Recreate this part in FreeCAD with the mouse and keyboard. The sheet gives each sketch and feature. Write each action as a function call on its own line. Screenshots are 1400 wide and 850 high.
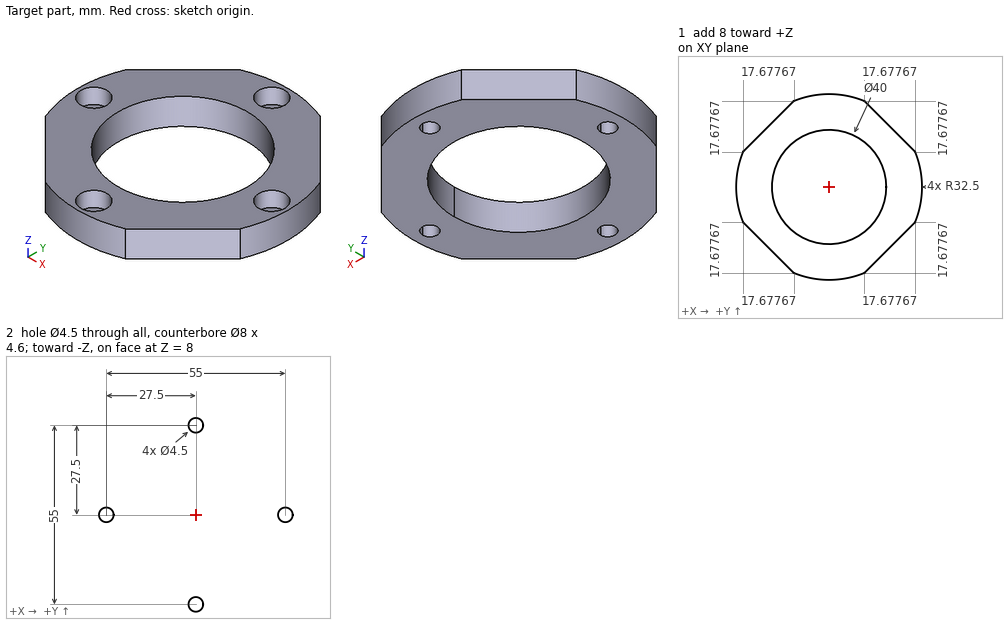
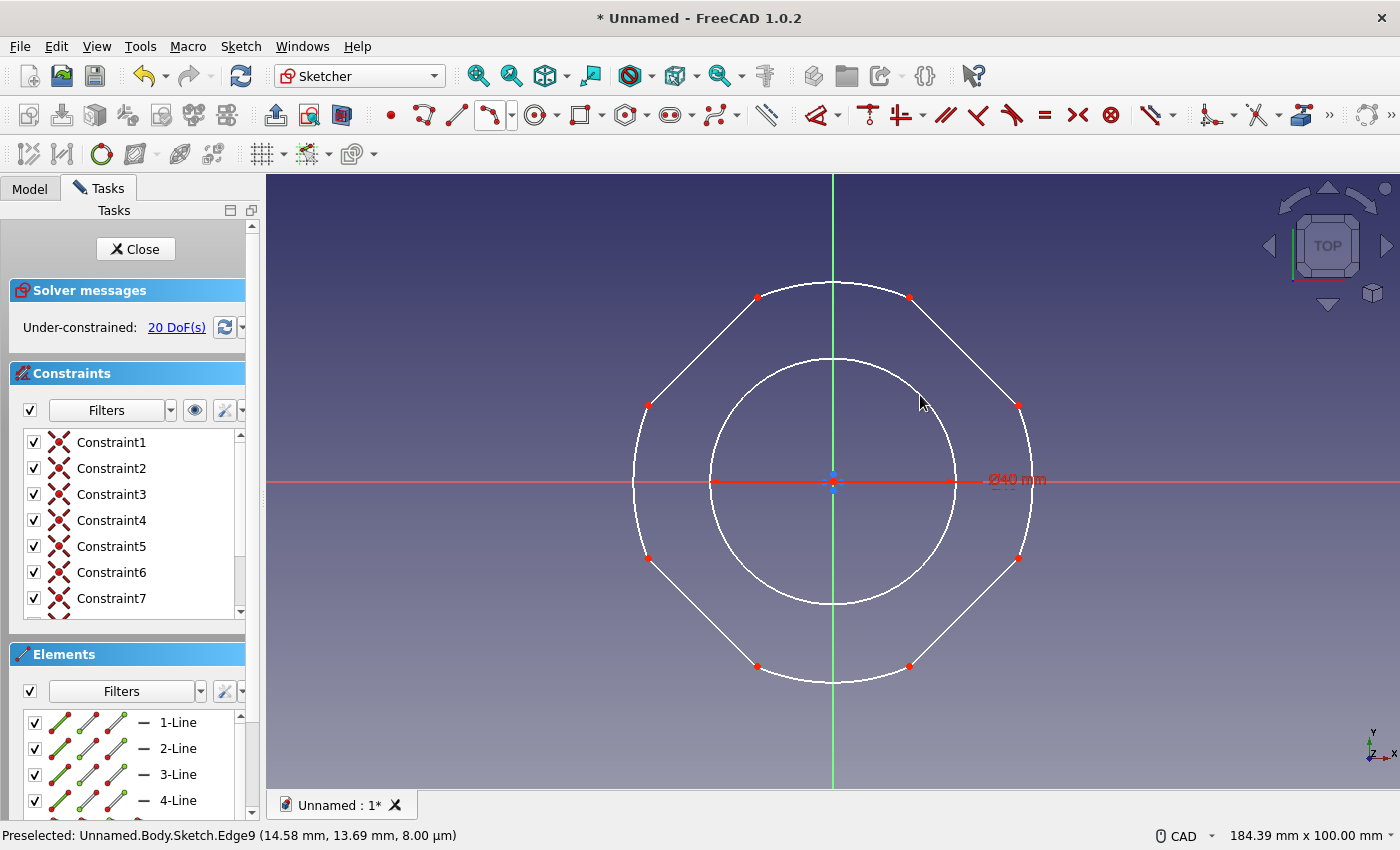
click(920, 394)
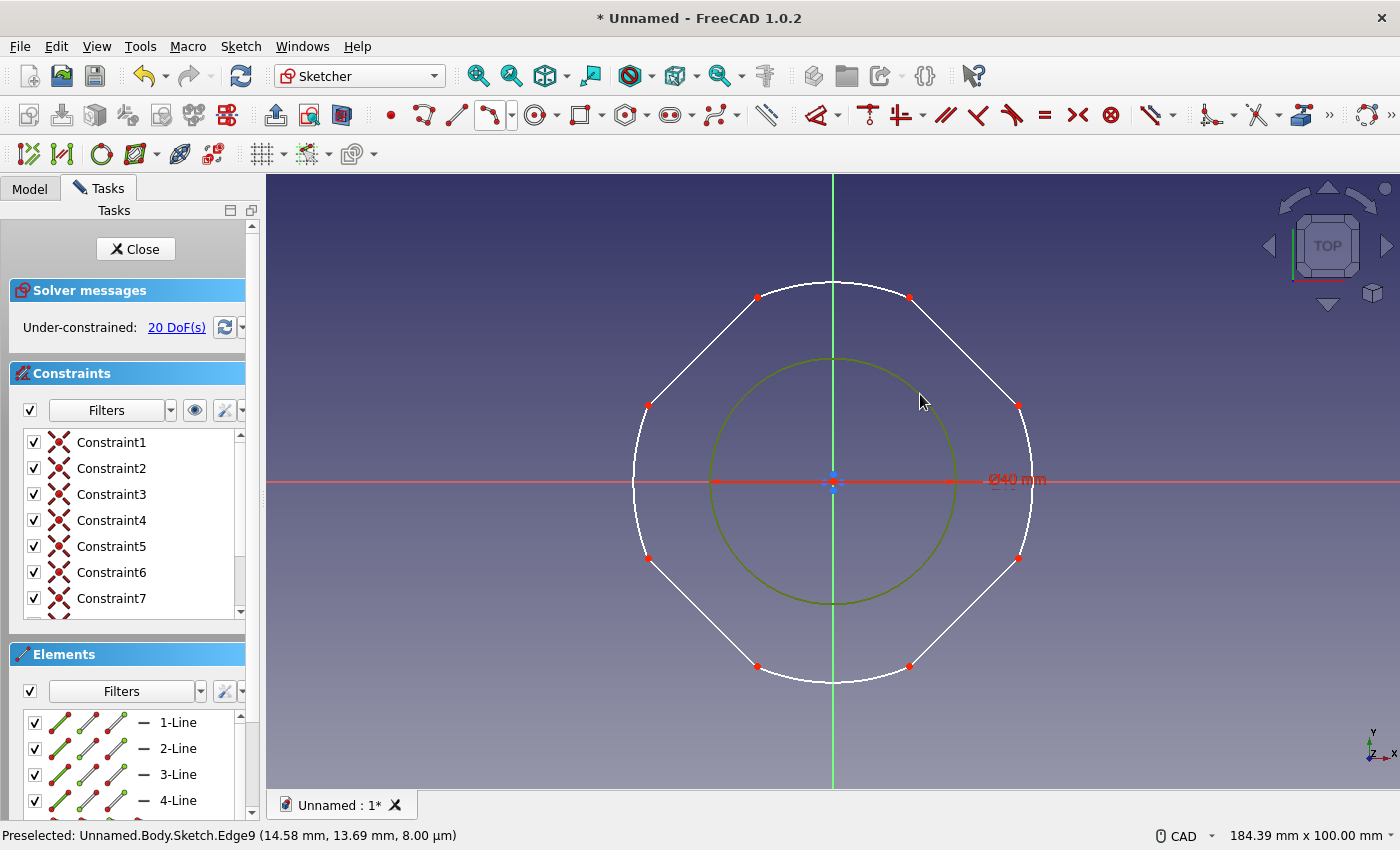
click(802, 680)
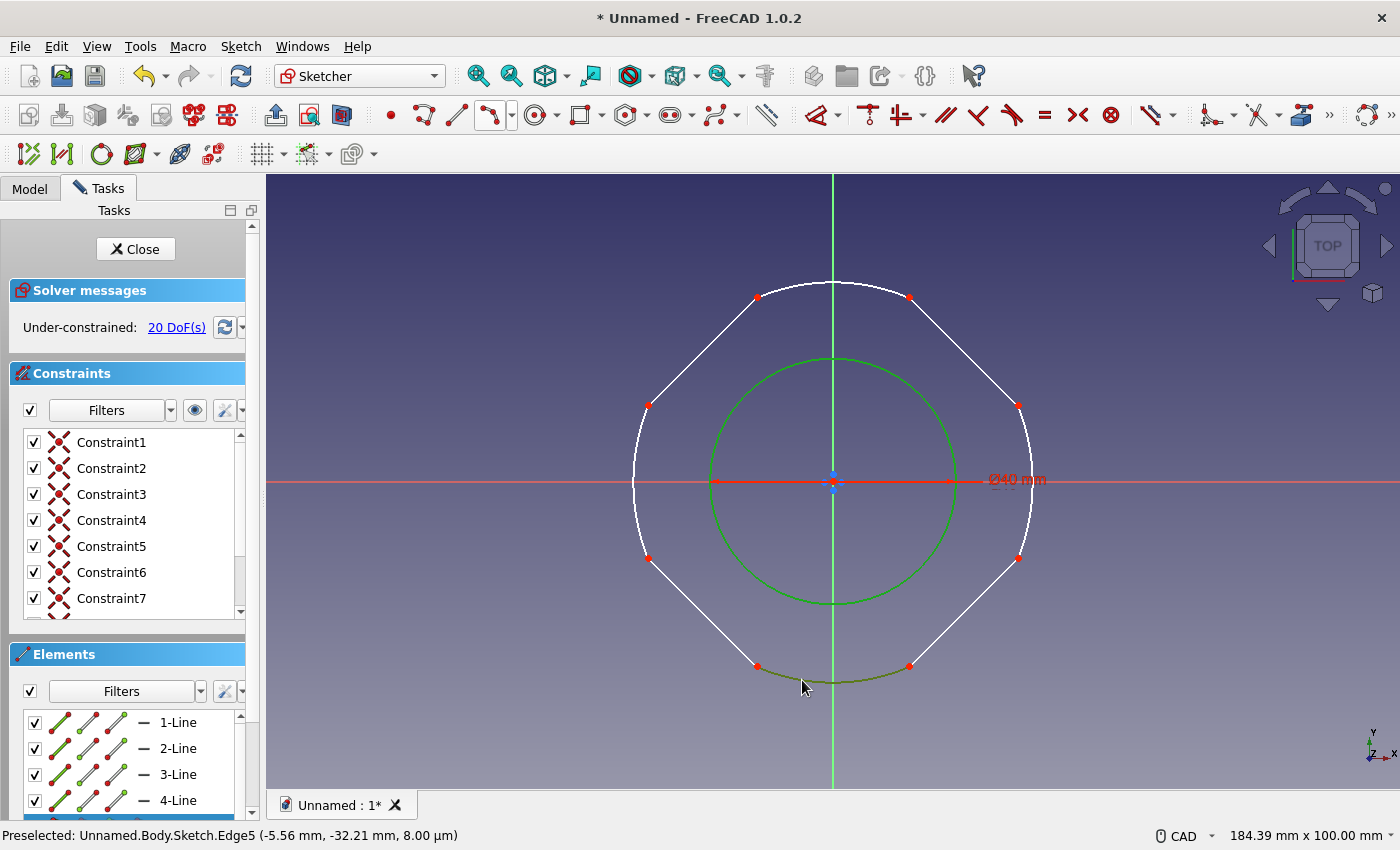
click(868, 116)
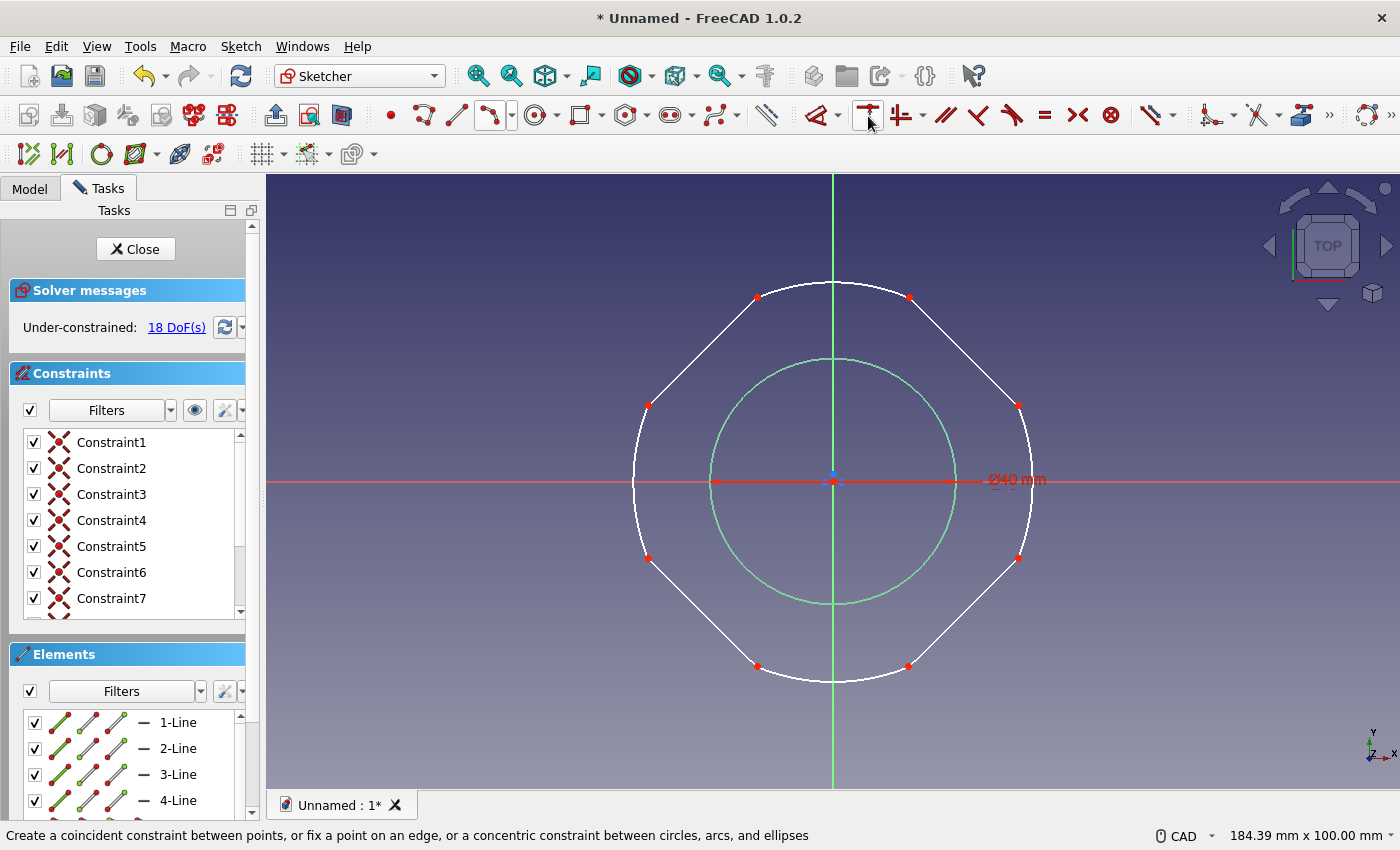
click(920, 394)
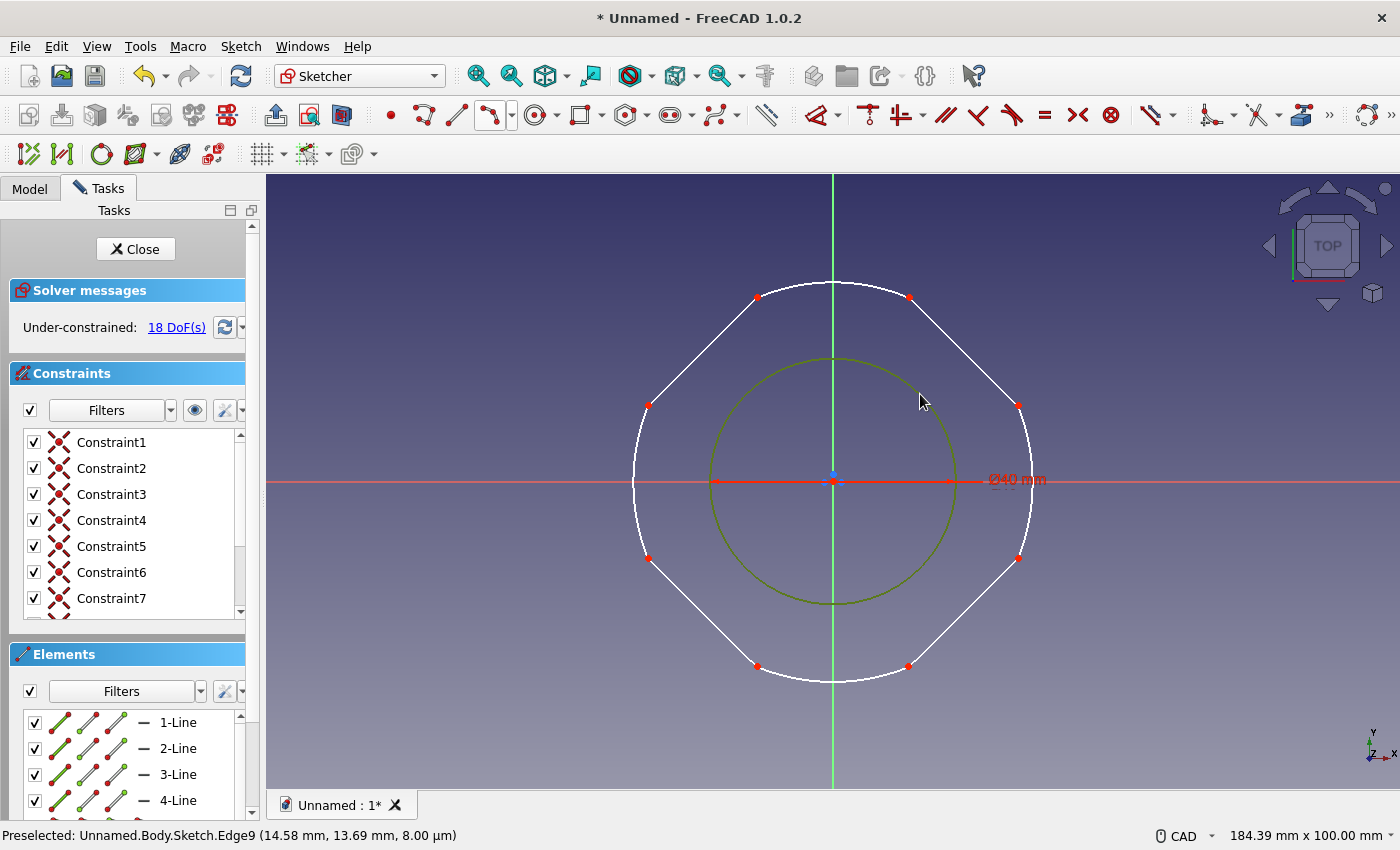
click(1030, 514)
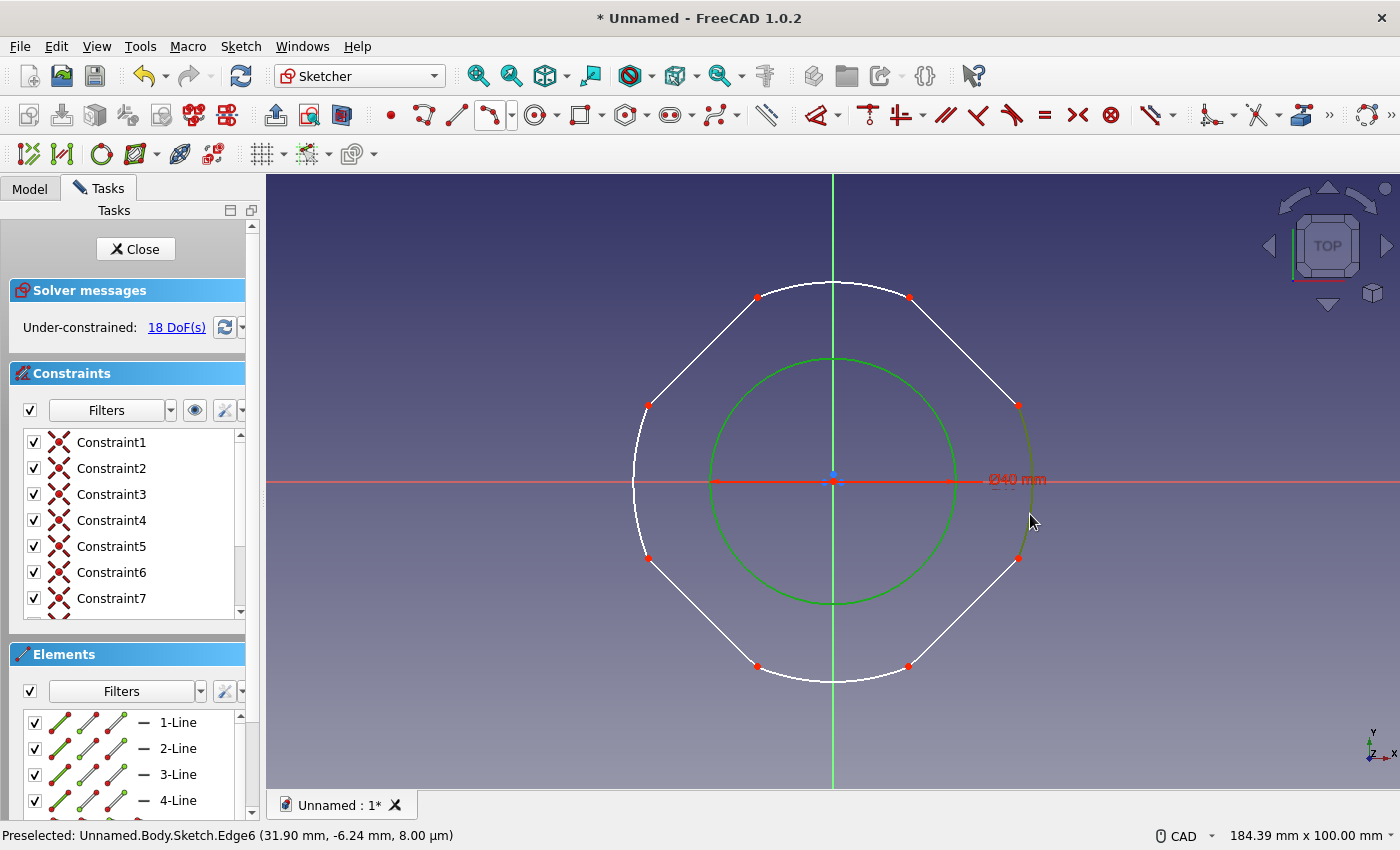
click(868, 116)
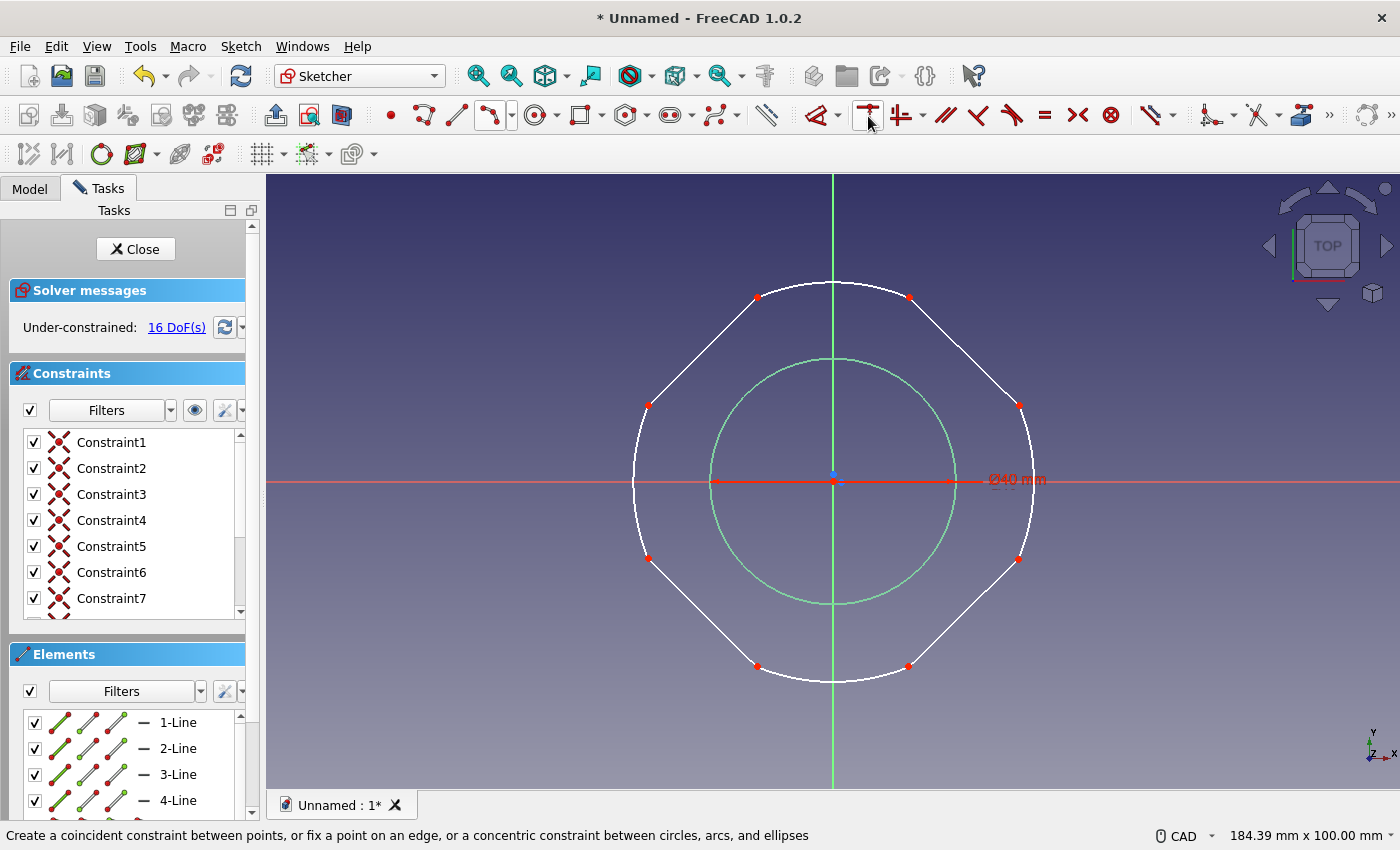
click(920, 394)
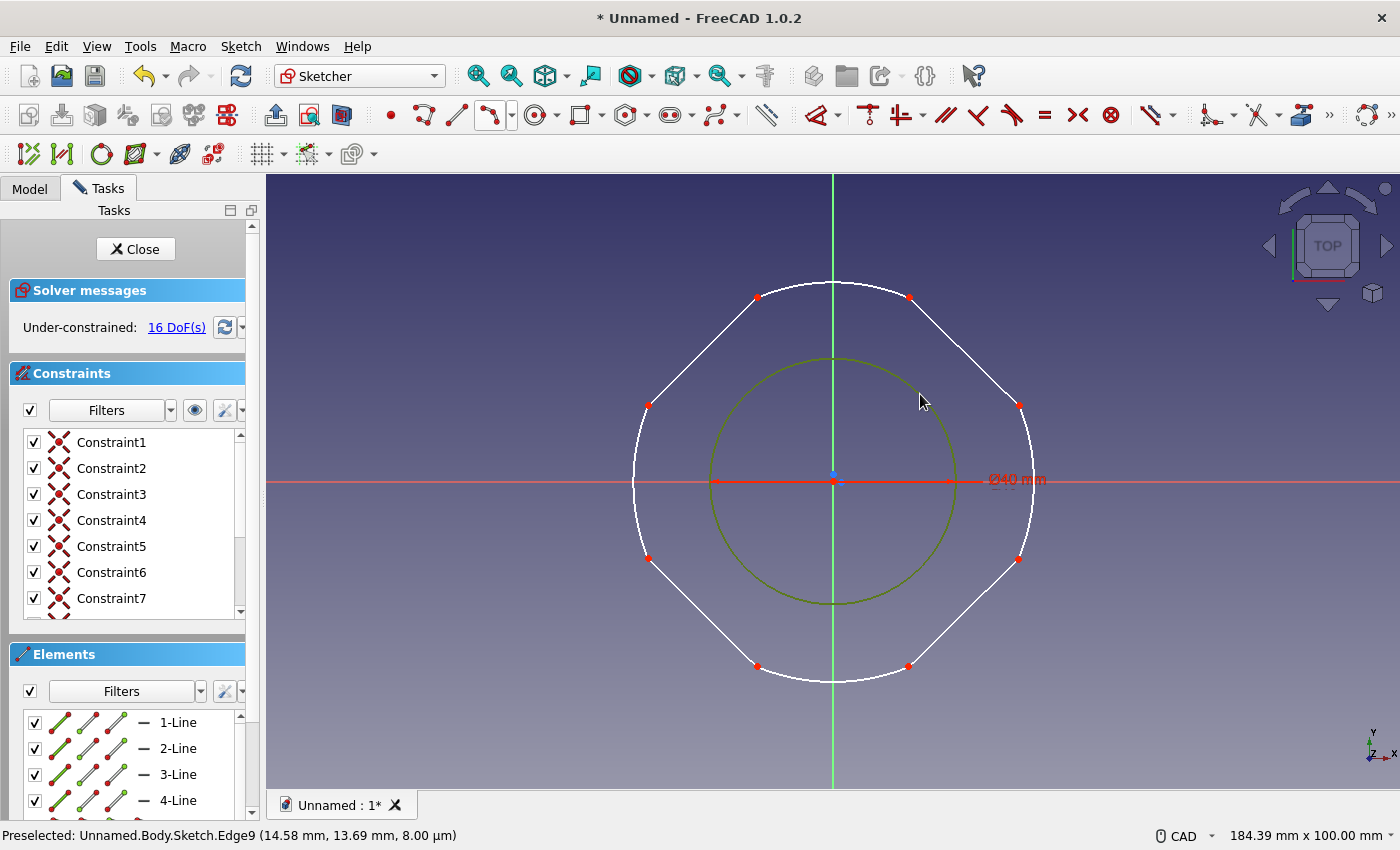
click(864, 285)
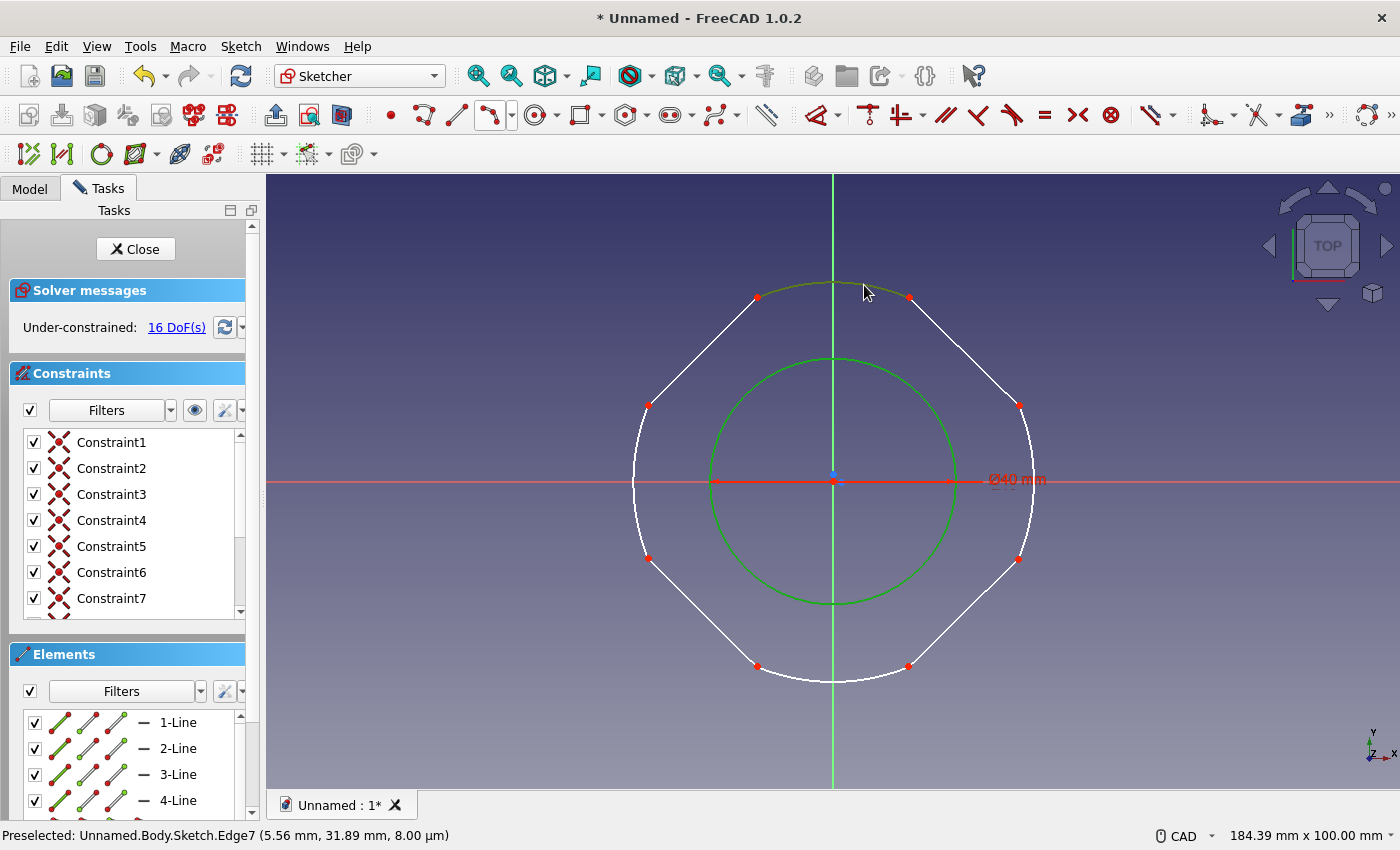
click(868, 116)